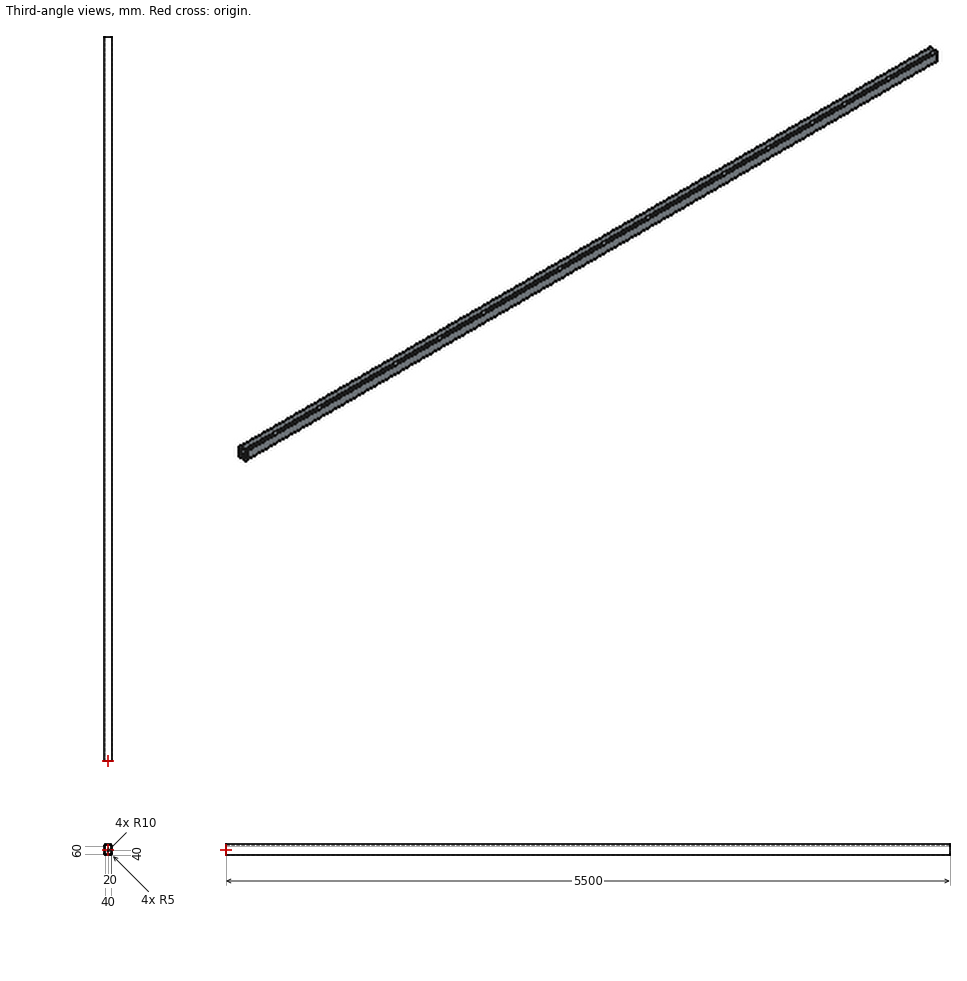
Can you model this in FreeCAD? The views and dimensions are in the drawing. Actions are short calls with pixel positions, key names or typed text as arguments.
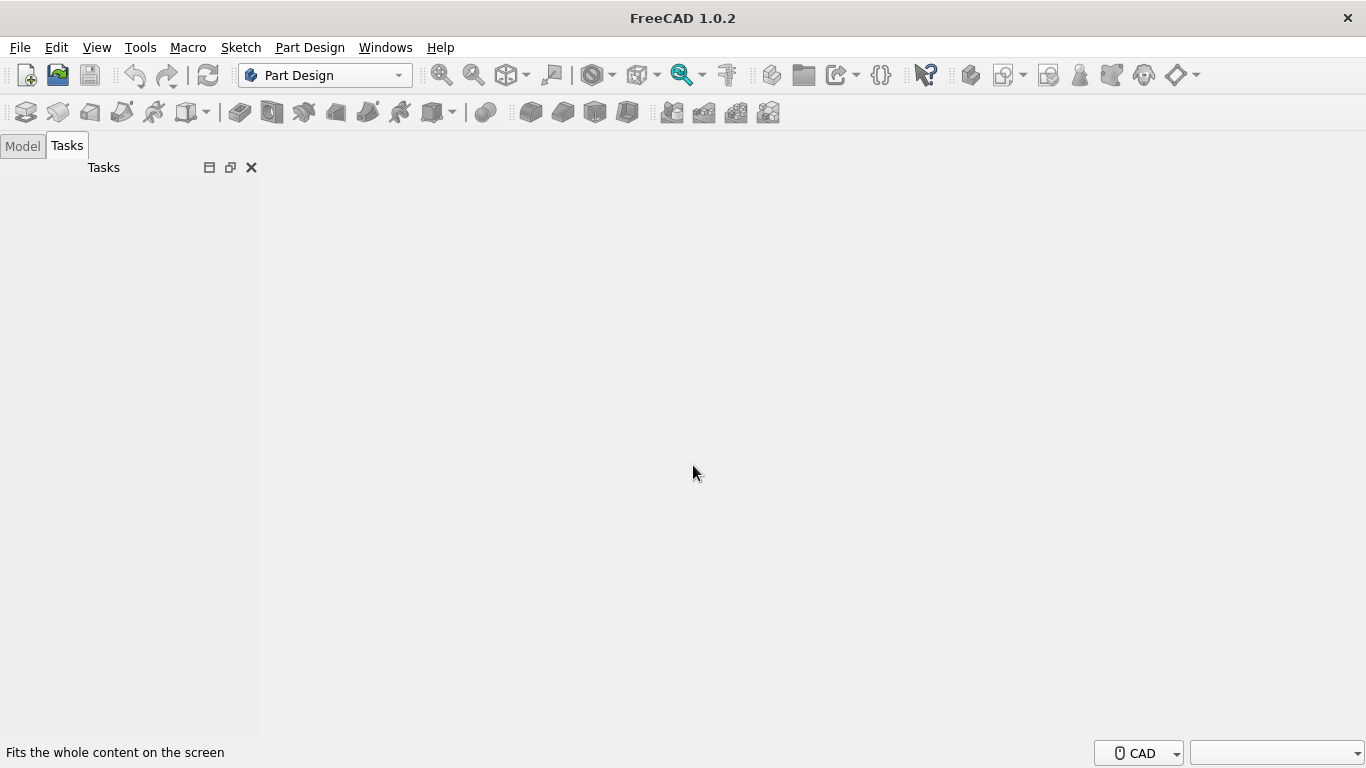
click(26, 76)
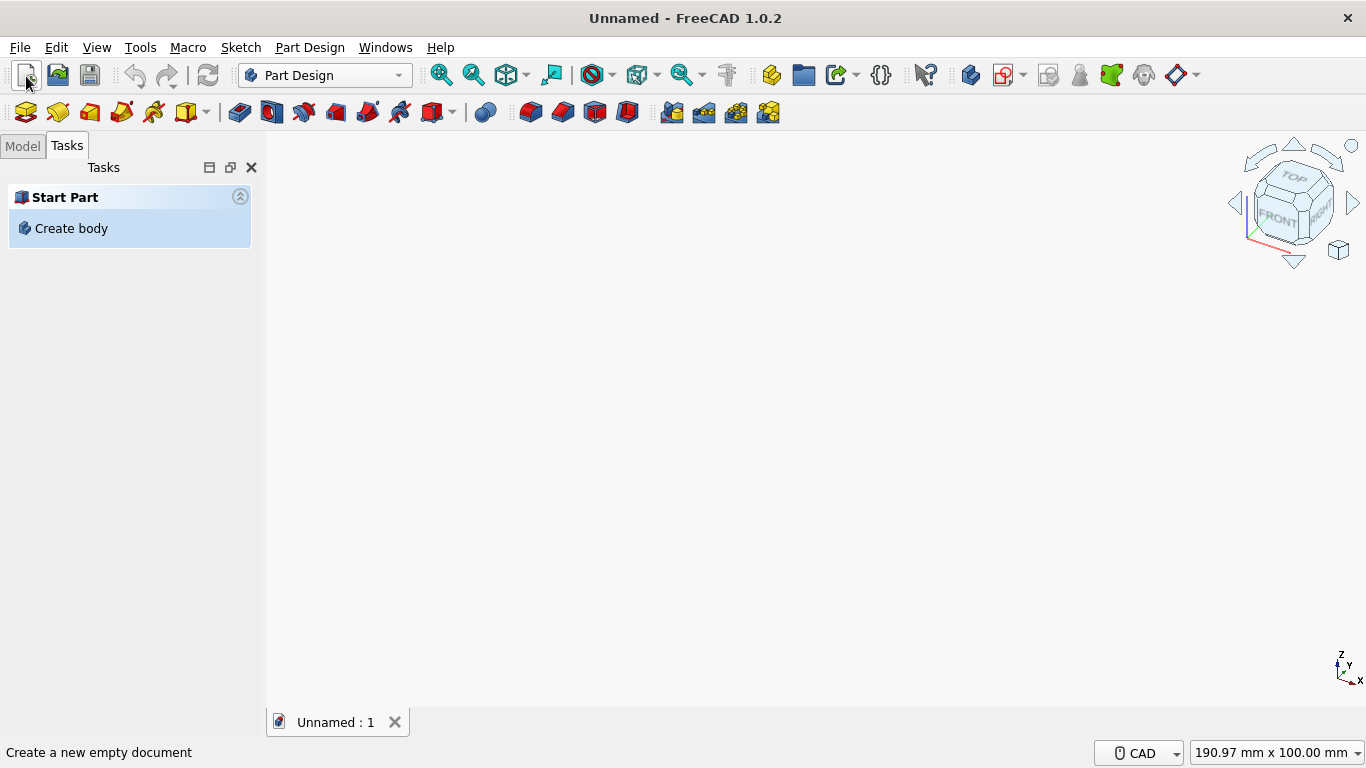
click(1004, 76)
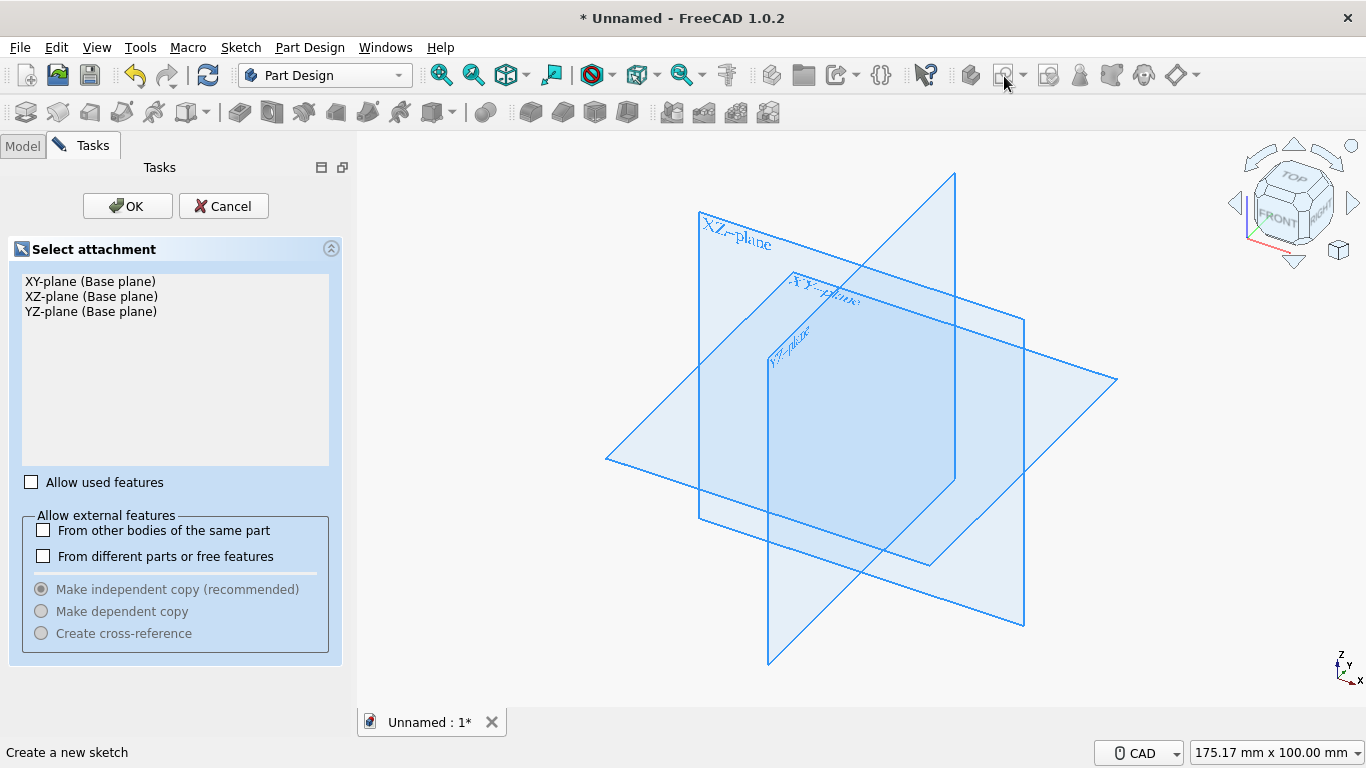
click(82, 296)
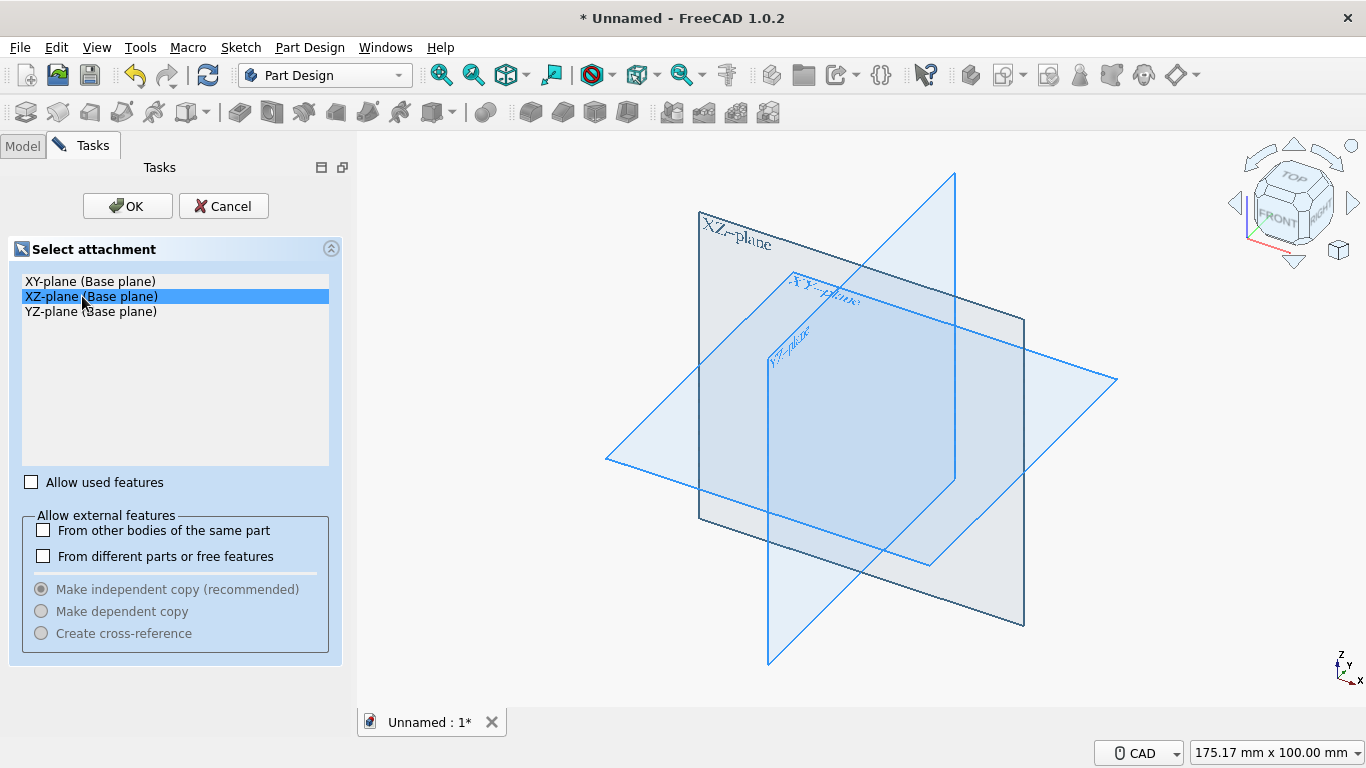
click(128, 206)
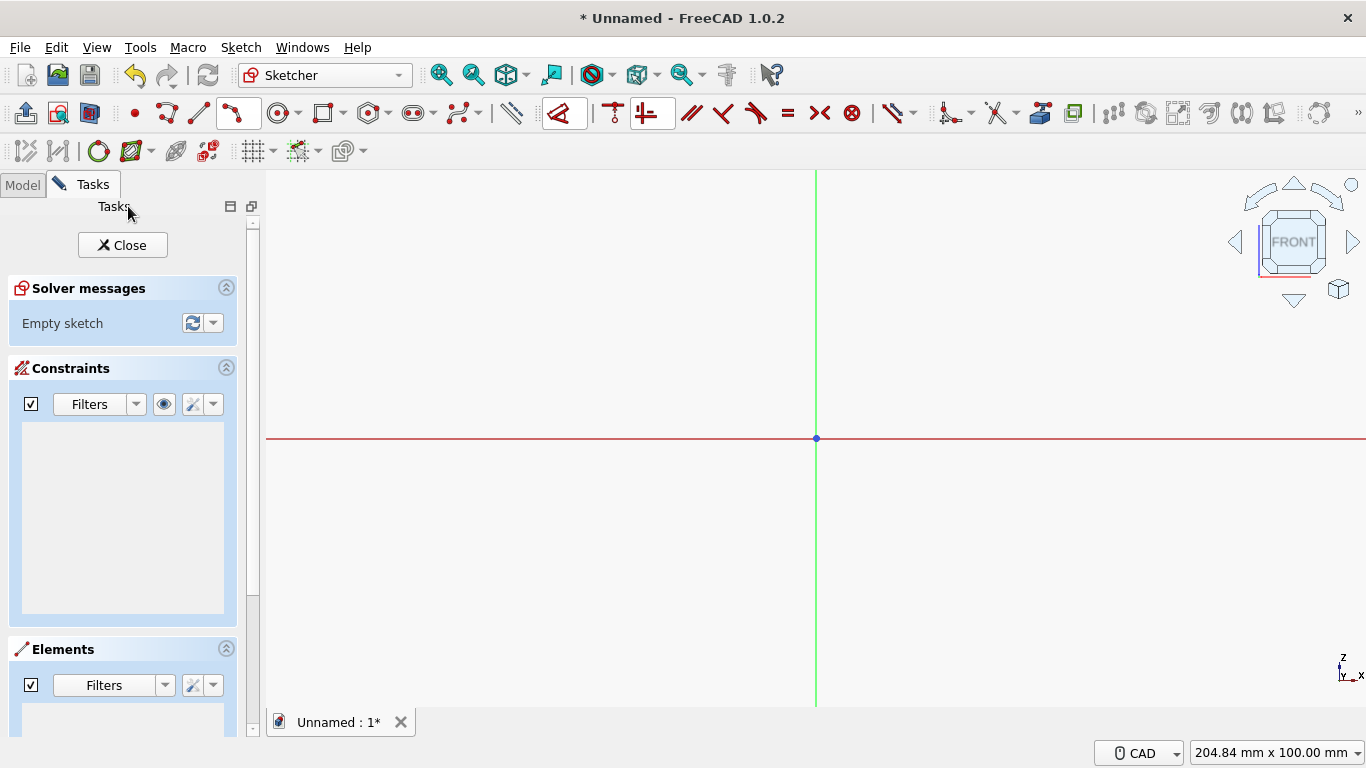
click(200, 114)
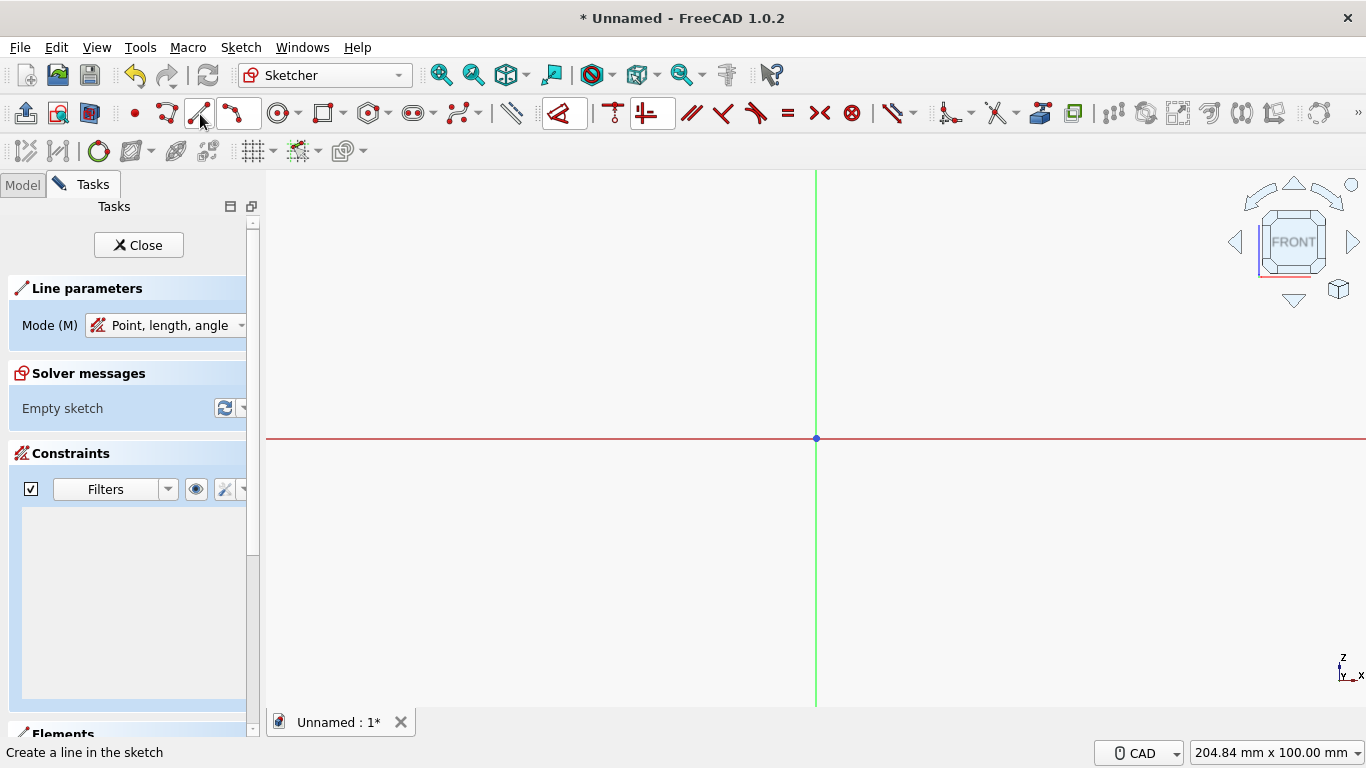
click(923, 653)
click(709, 653)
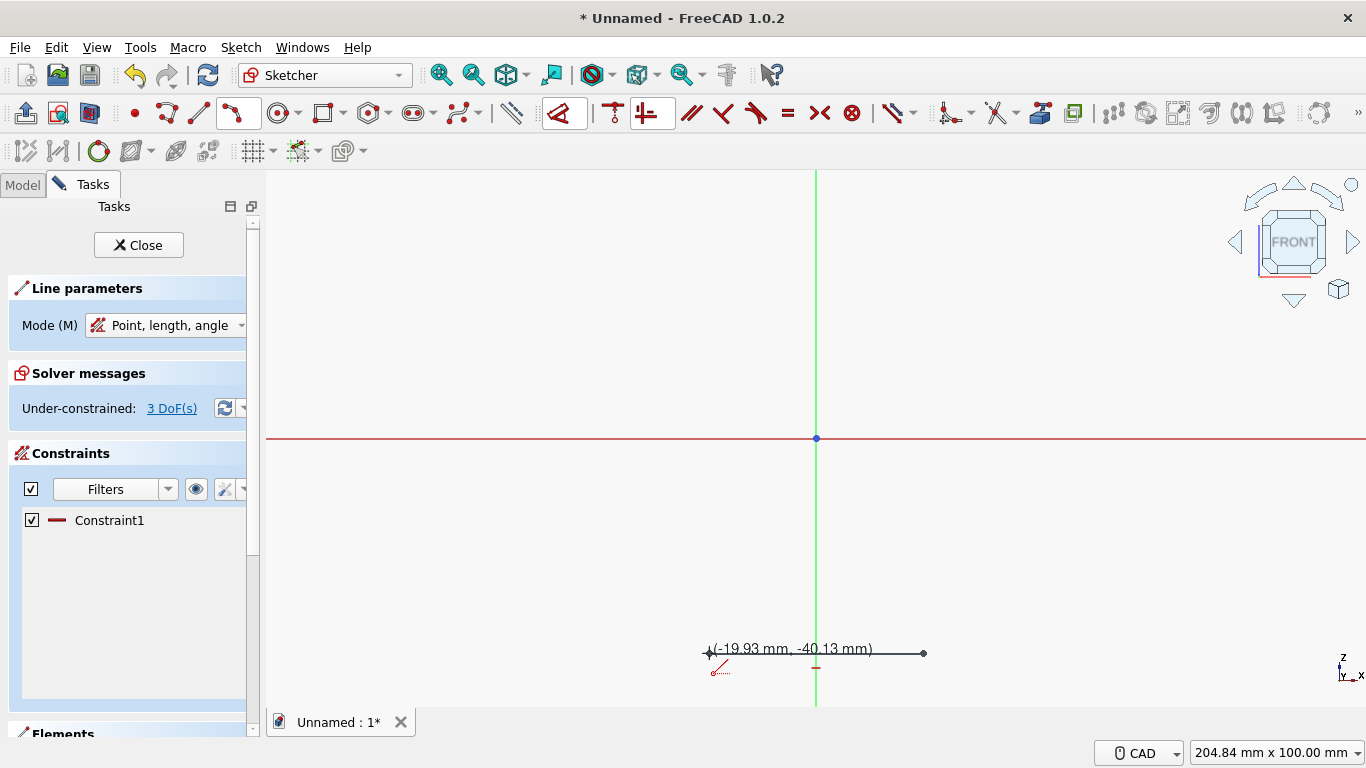
click(655, 600)
click(655, 277)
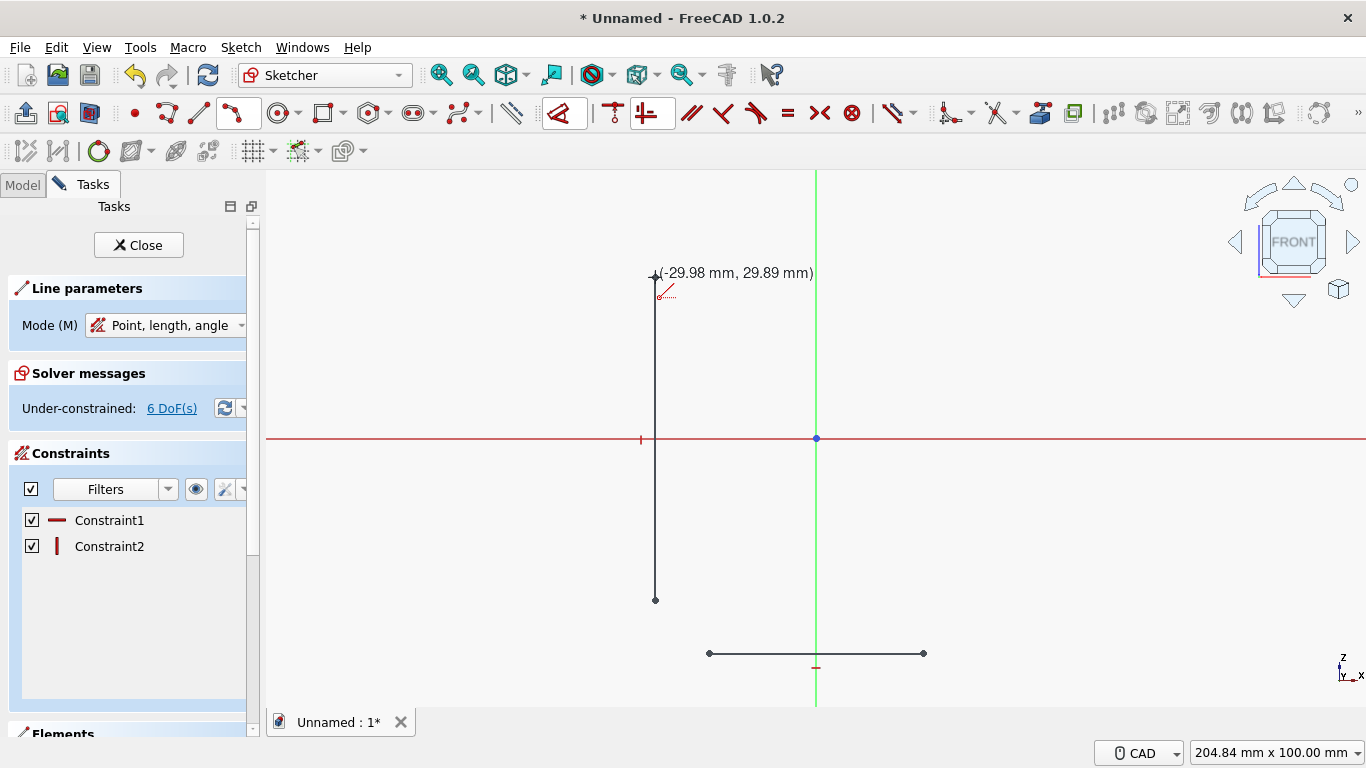
click(709, 224)
click(923, 224)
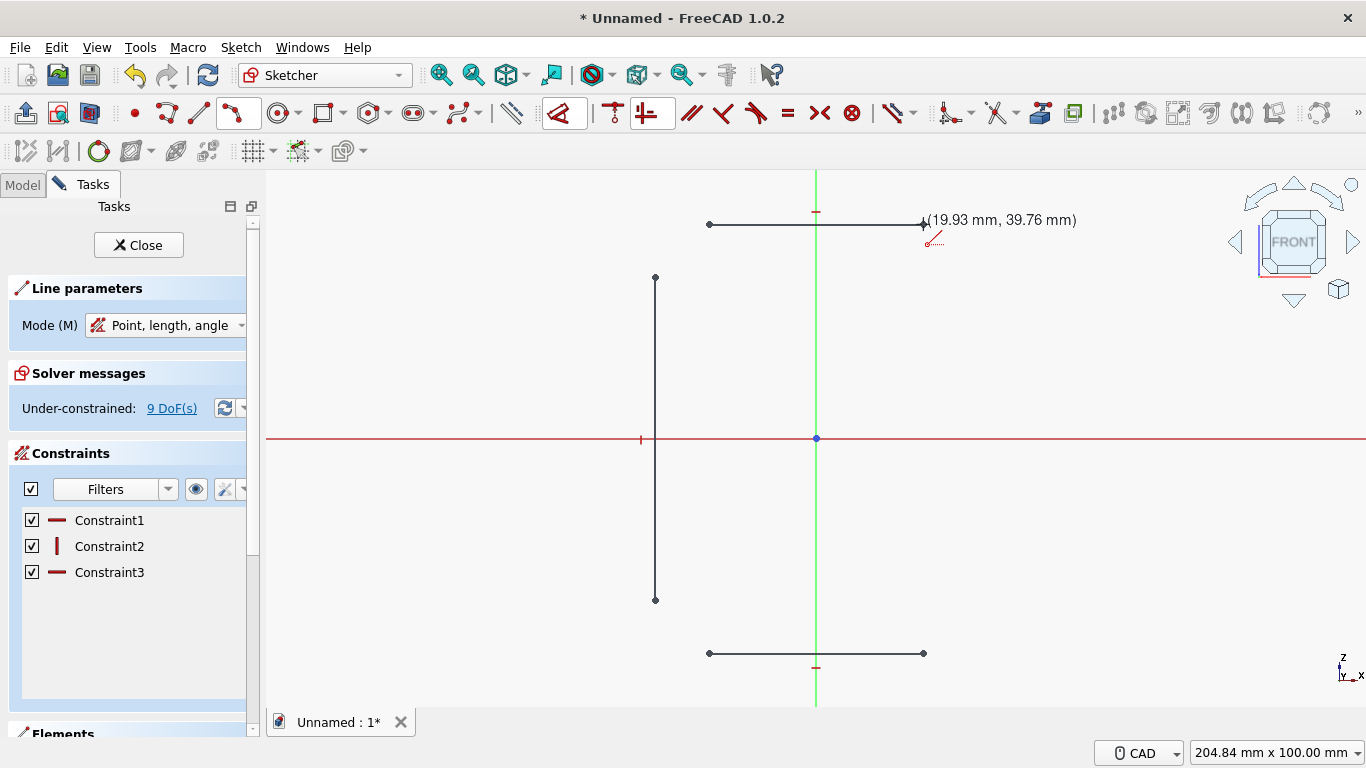
click(977, 277)
click(977, 600)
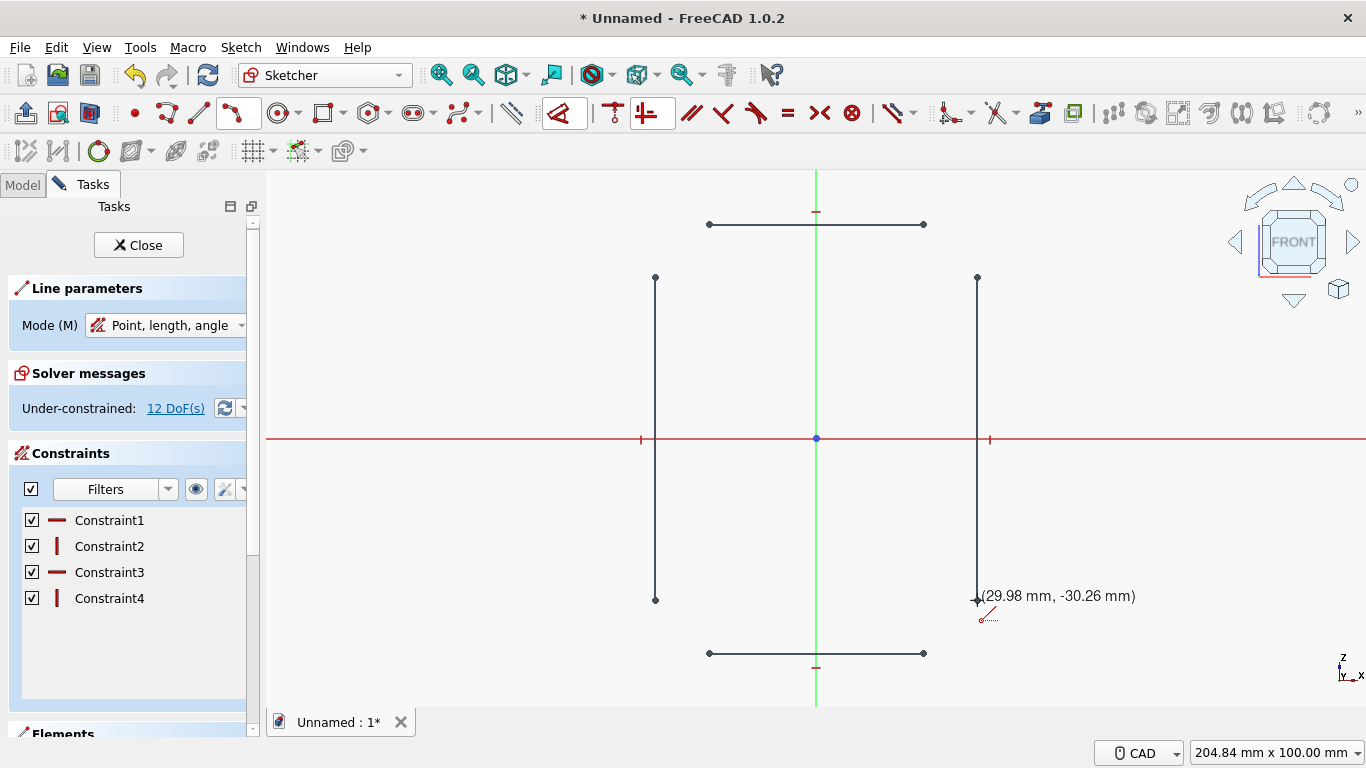
click(232, 114)